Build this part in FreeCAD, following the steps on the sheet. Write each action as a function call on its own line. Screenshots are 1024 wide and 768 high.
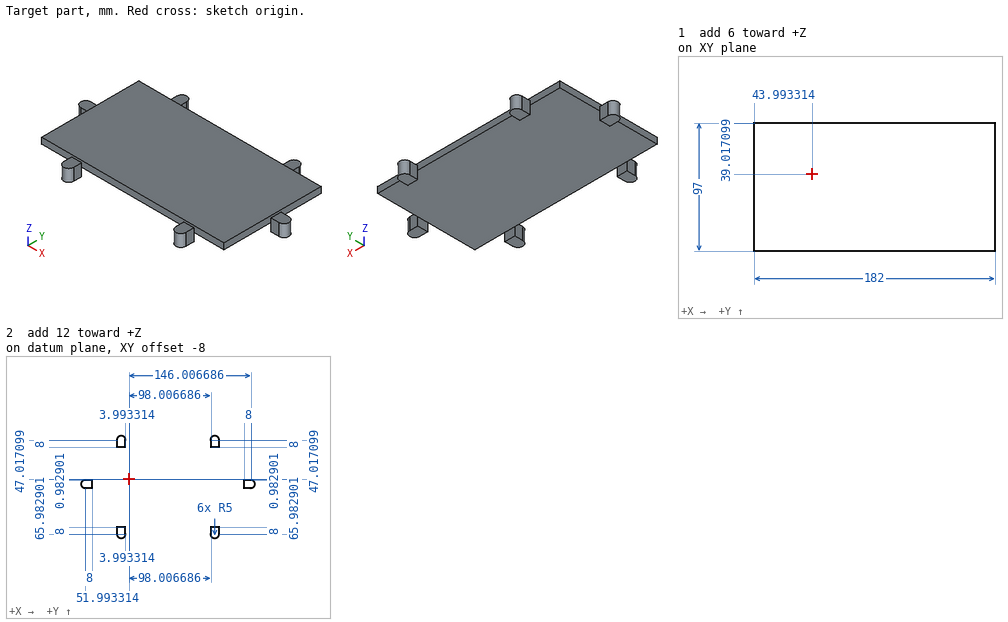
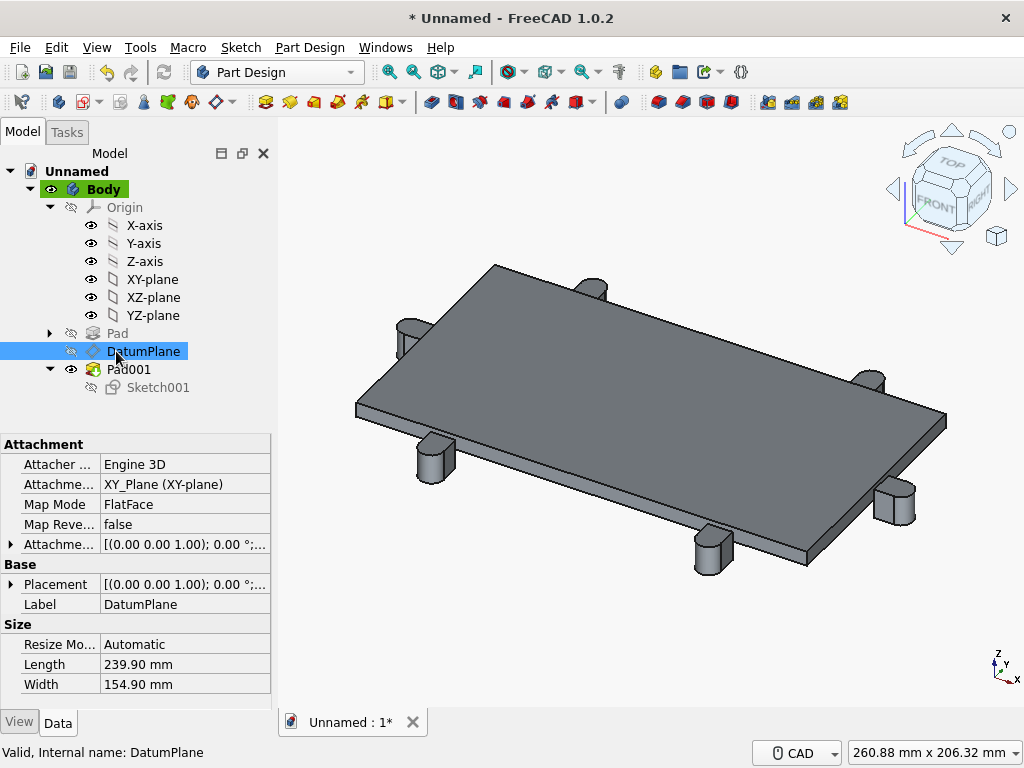
key(0)